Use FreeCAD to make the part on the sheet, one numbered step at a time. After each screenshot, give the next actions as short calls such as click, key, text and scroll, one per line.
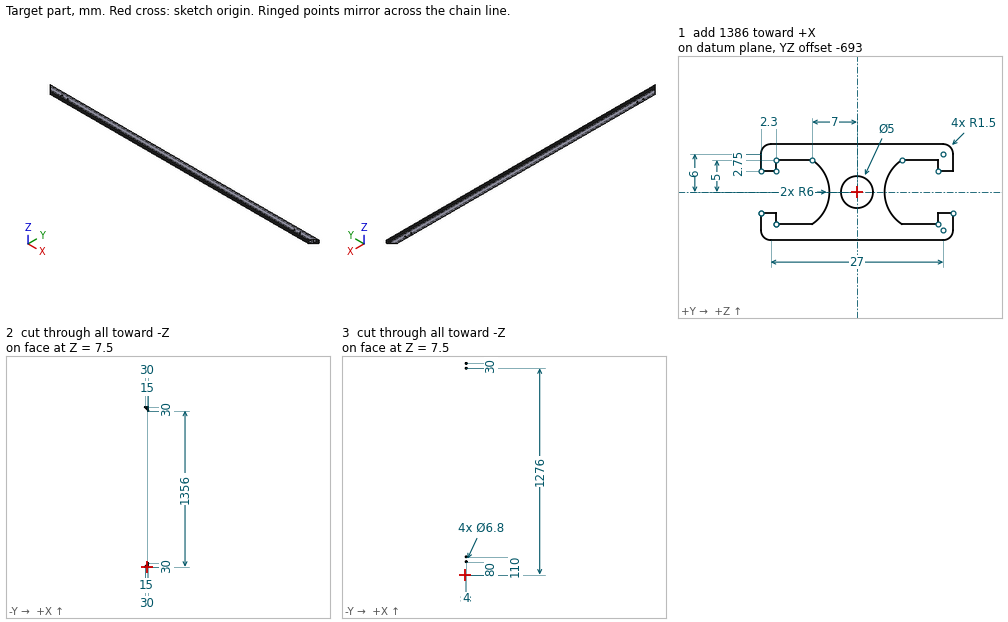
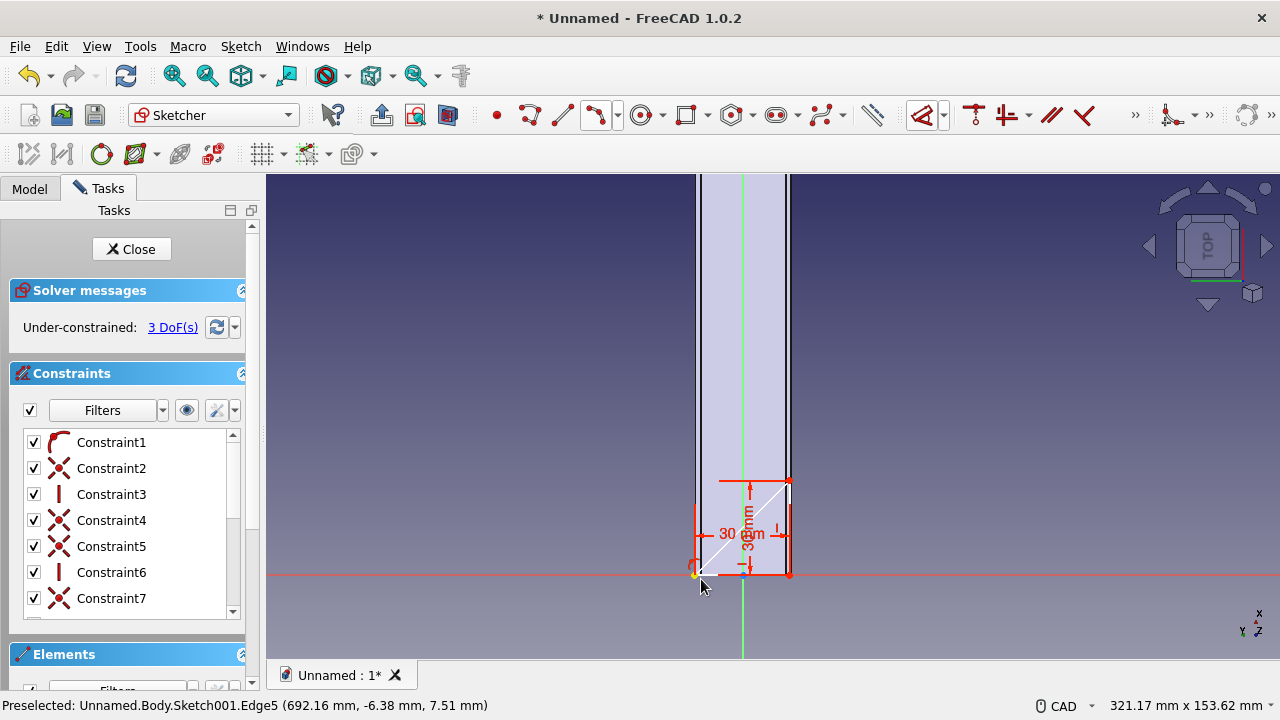
click(695, 575)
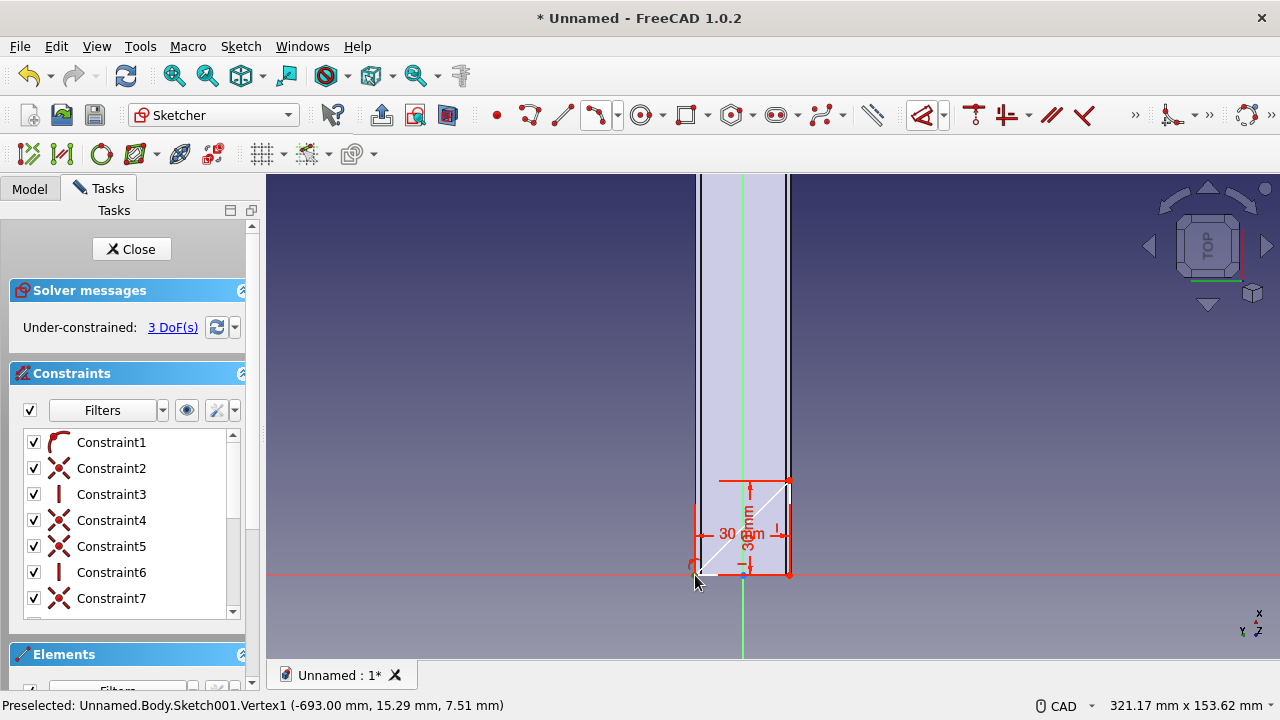
click(944, 116)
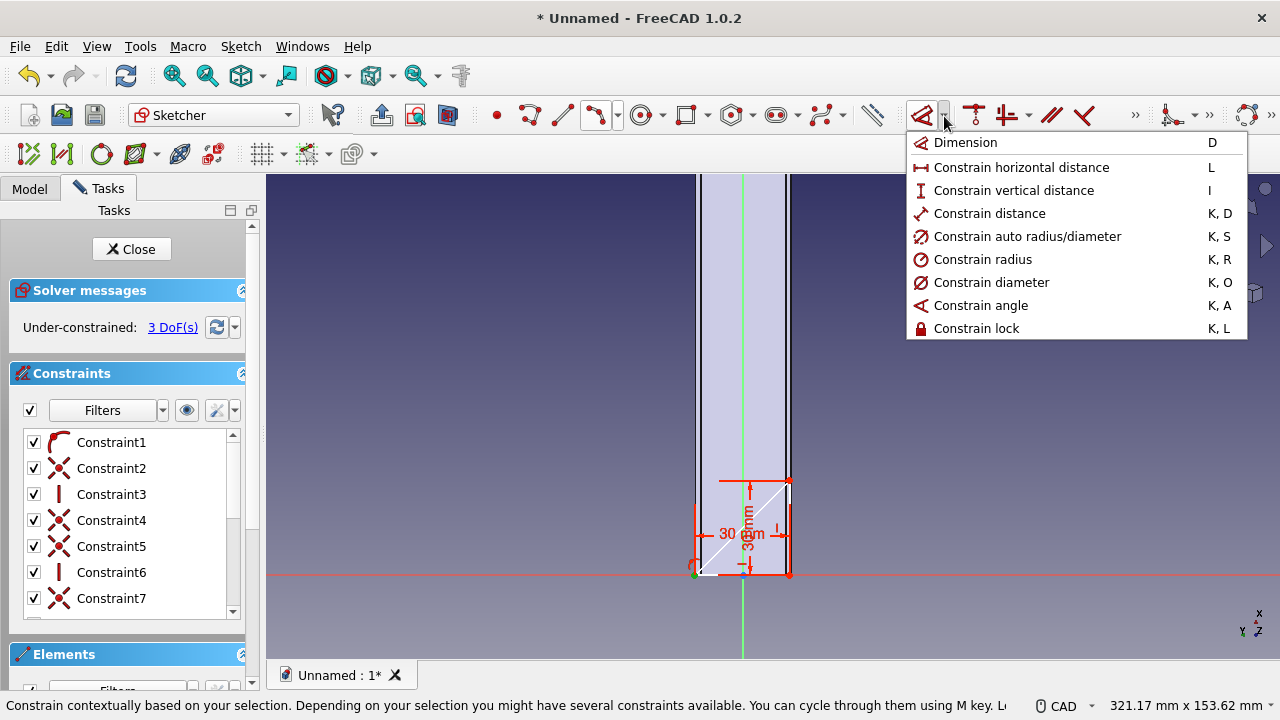
click(1077, 168)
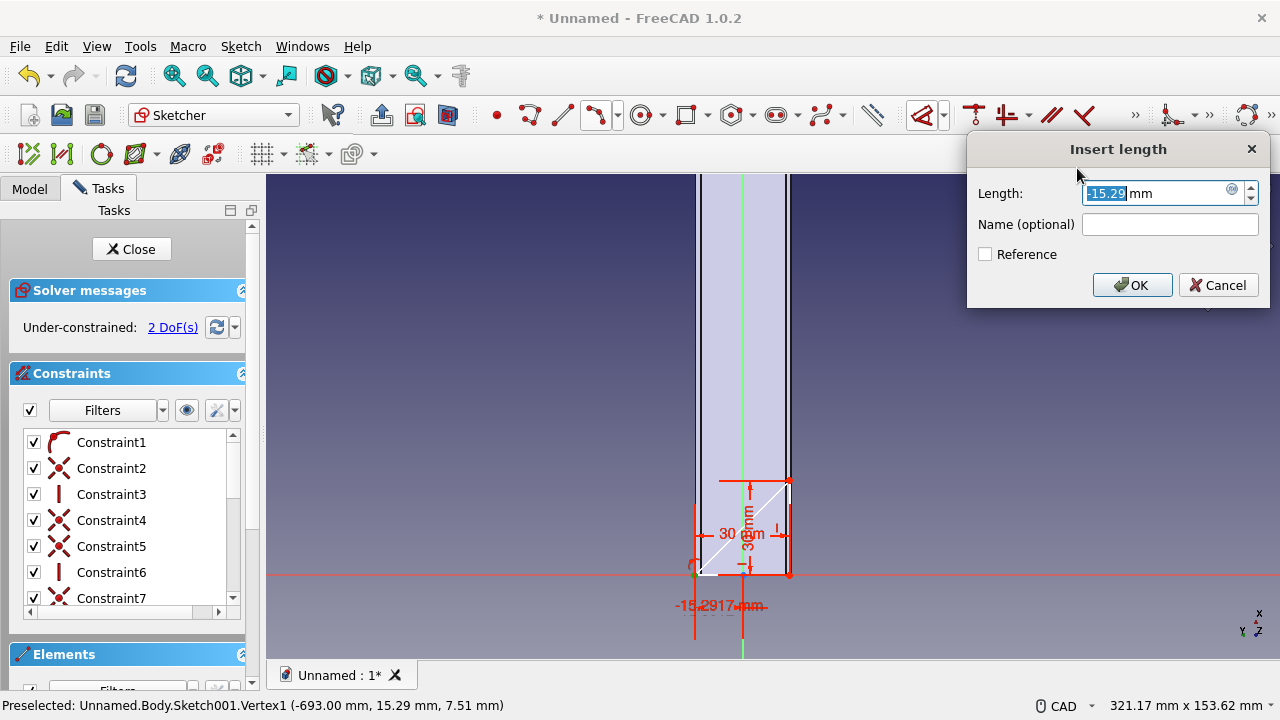
text(-15)
key(Return)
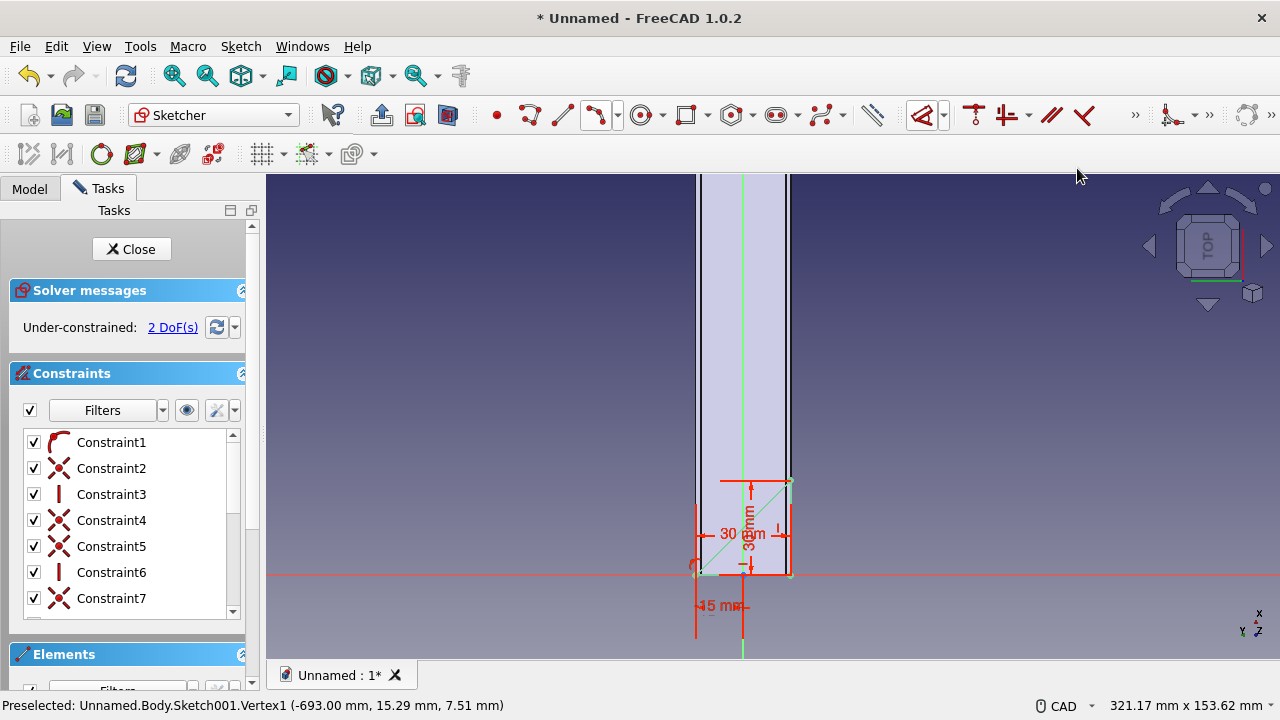
scroll(701, 579, down, 13)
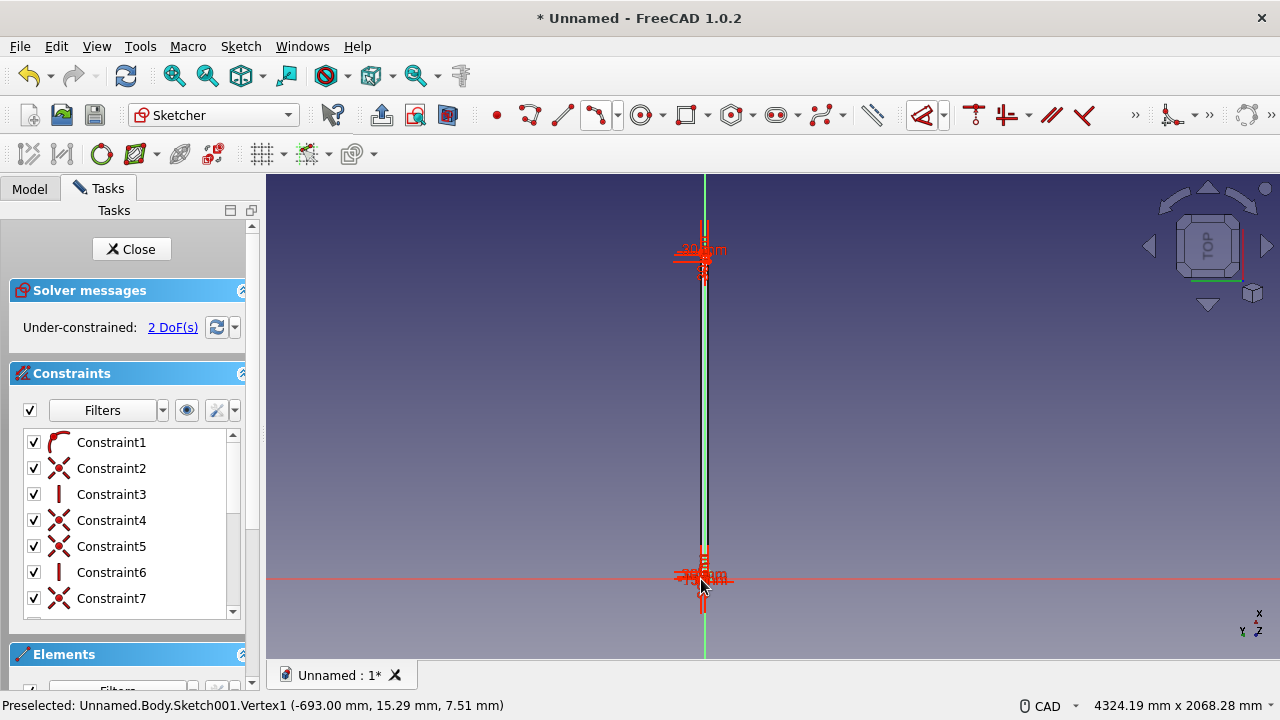
scroll(708, 262, up, 13)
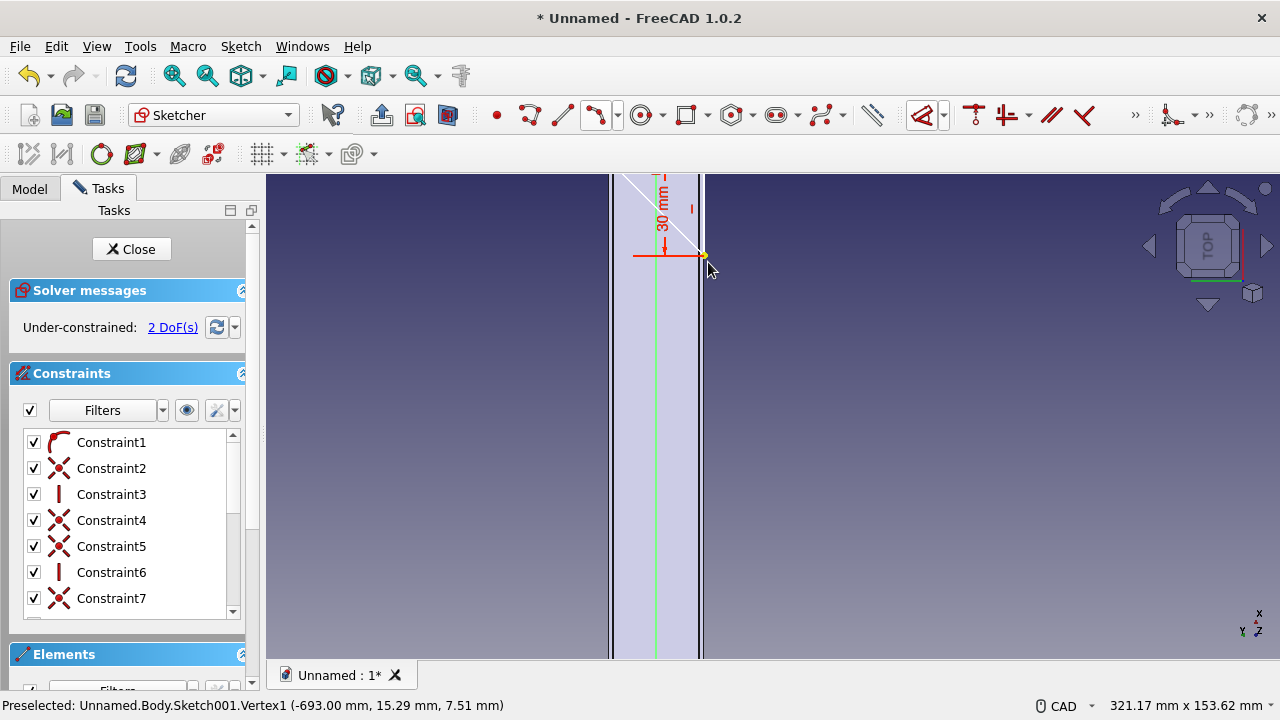
click(704, 256)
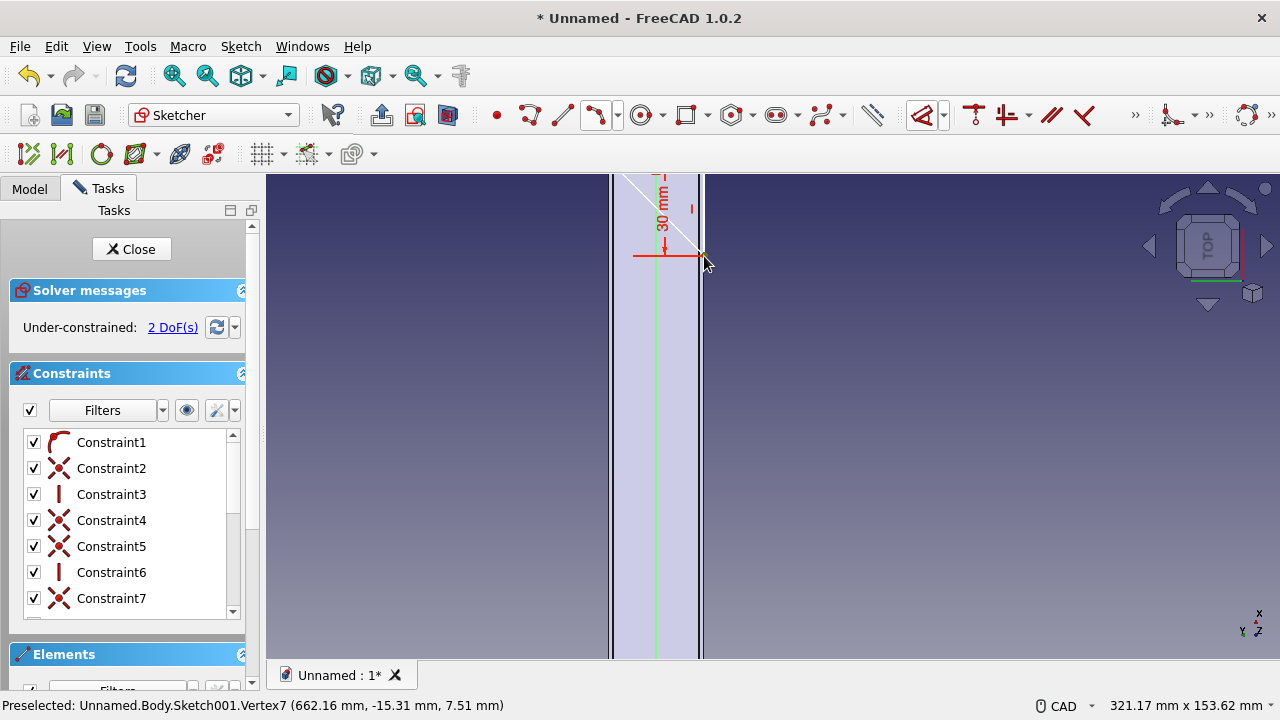
key(l)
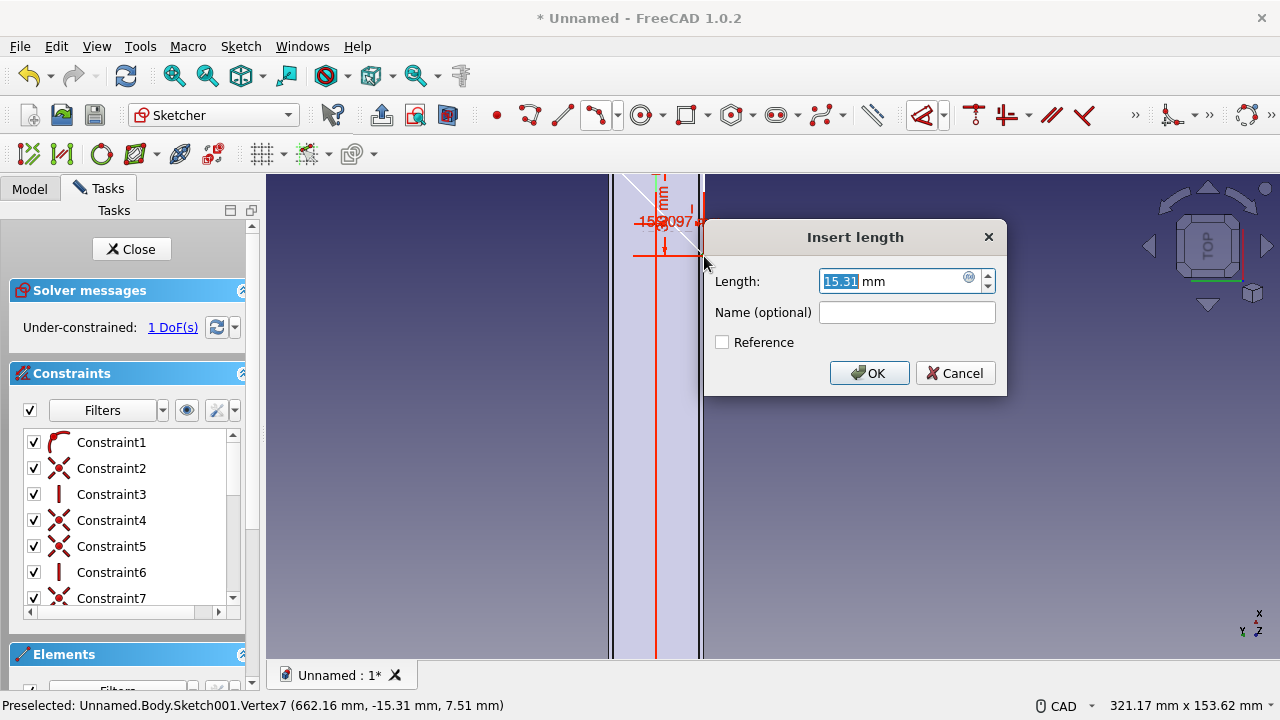
text(15)
key(Return)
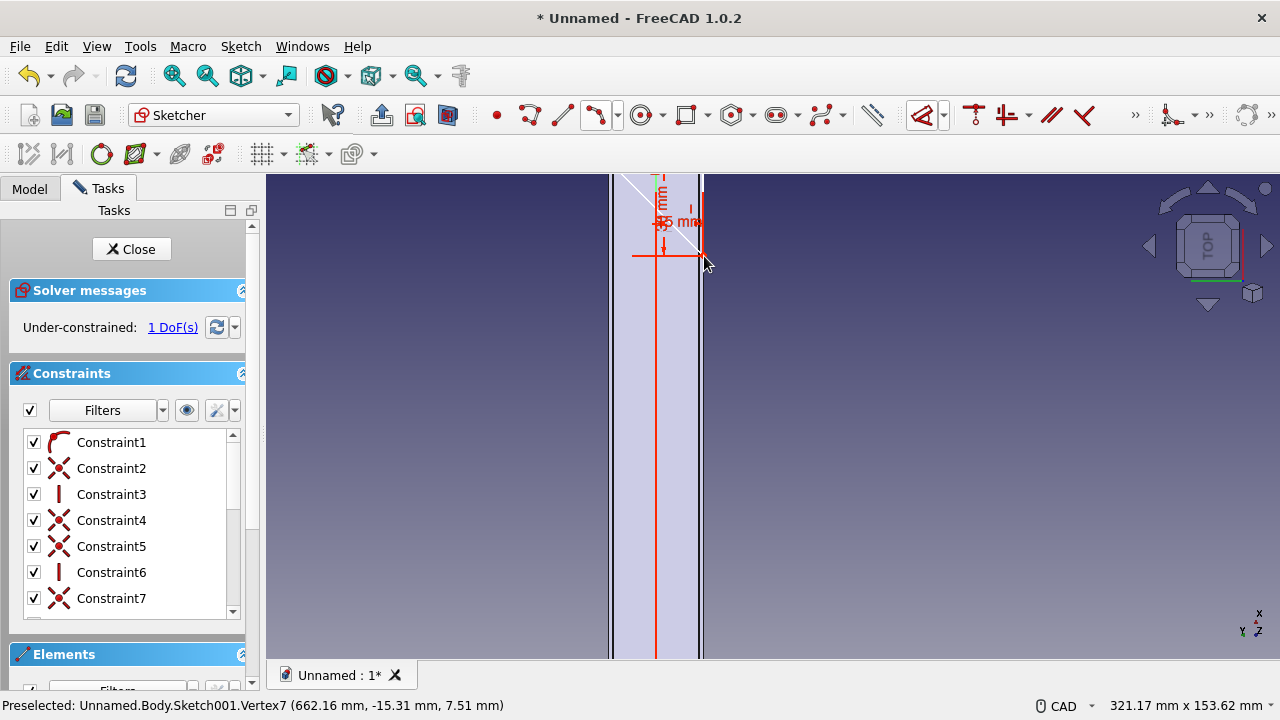
scroll(708, 262, down, 13)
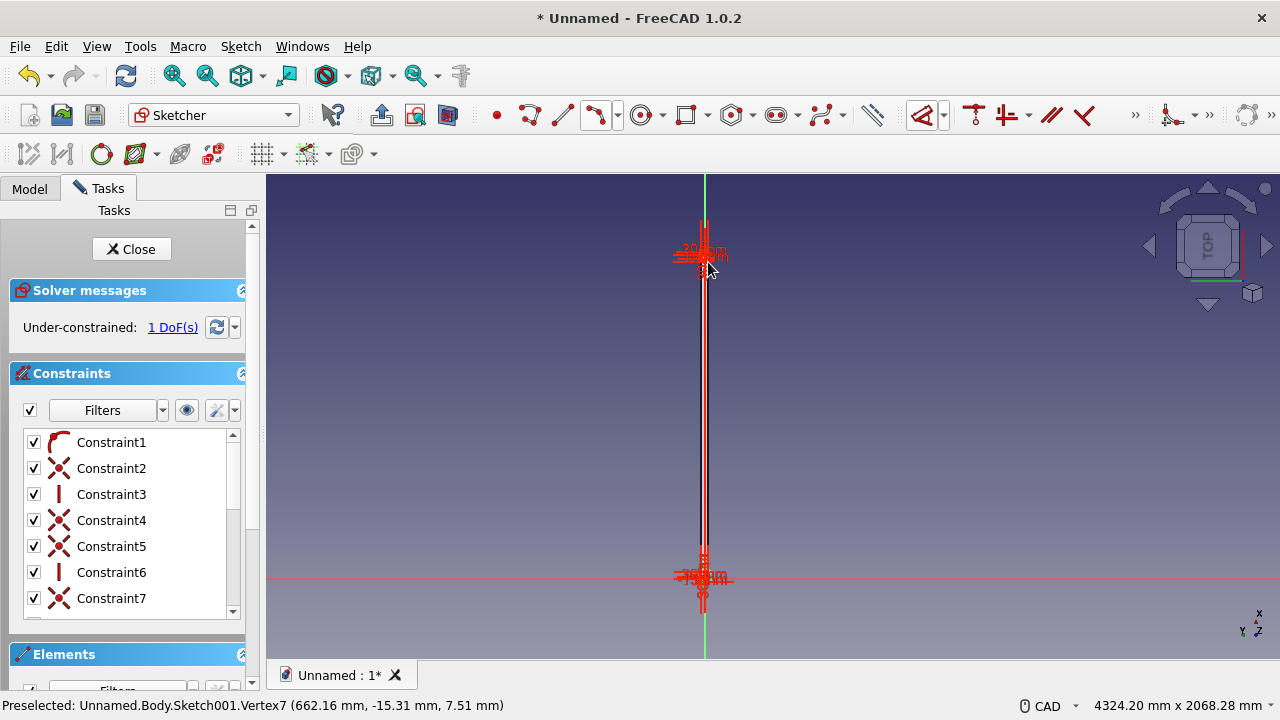
scroll(708, 262, up, 3)